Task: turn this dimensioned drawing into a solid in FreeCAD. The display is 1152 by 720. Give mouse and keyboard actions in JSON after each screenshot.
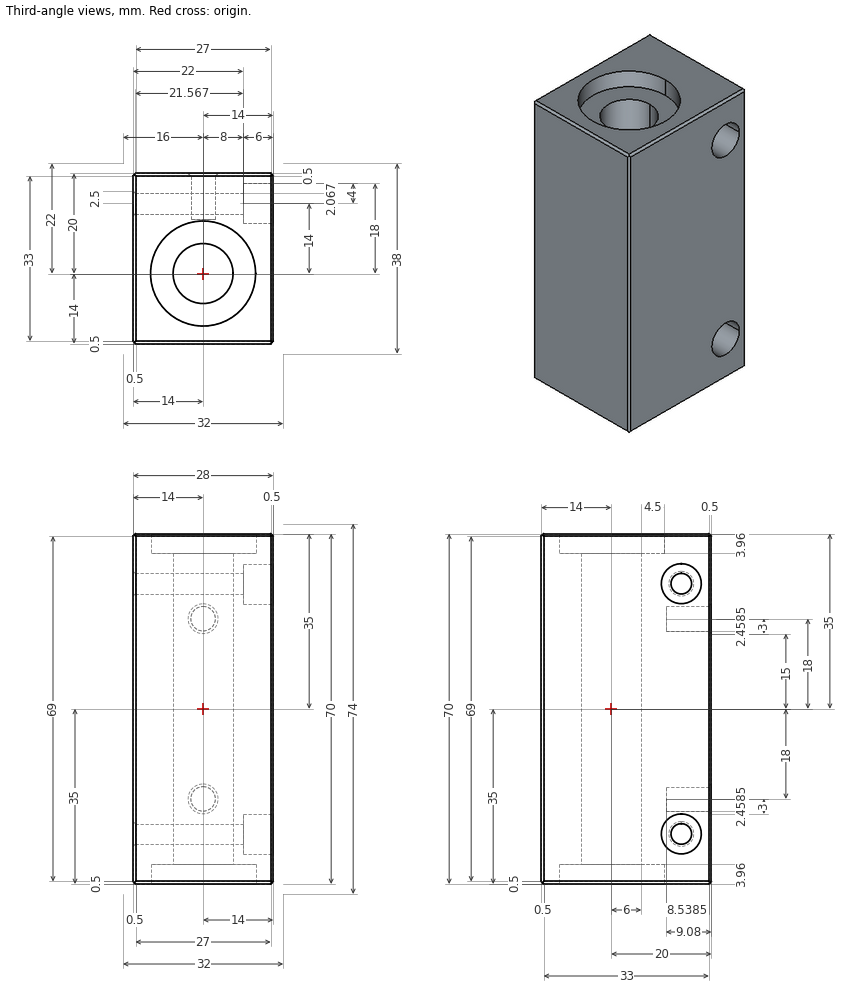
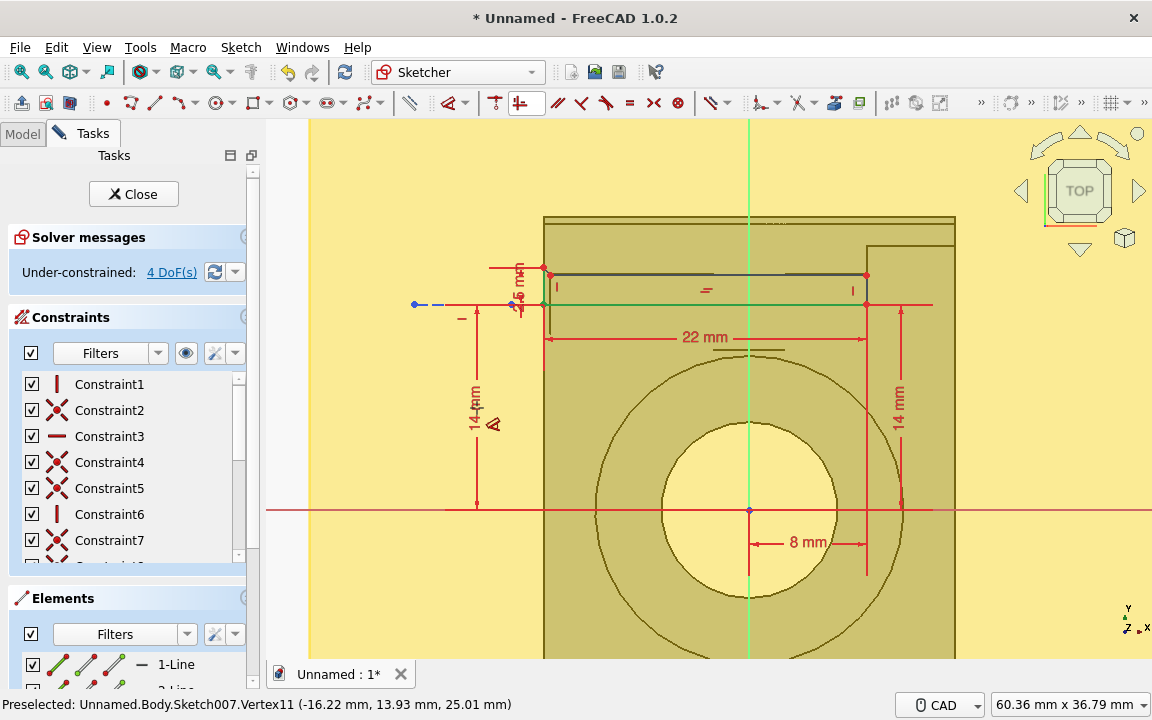
{"action": "scroll", "coordinate": [867, 293], "scroll_direction": "up", "scroll_amount": 2}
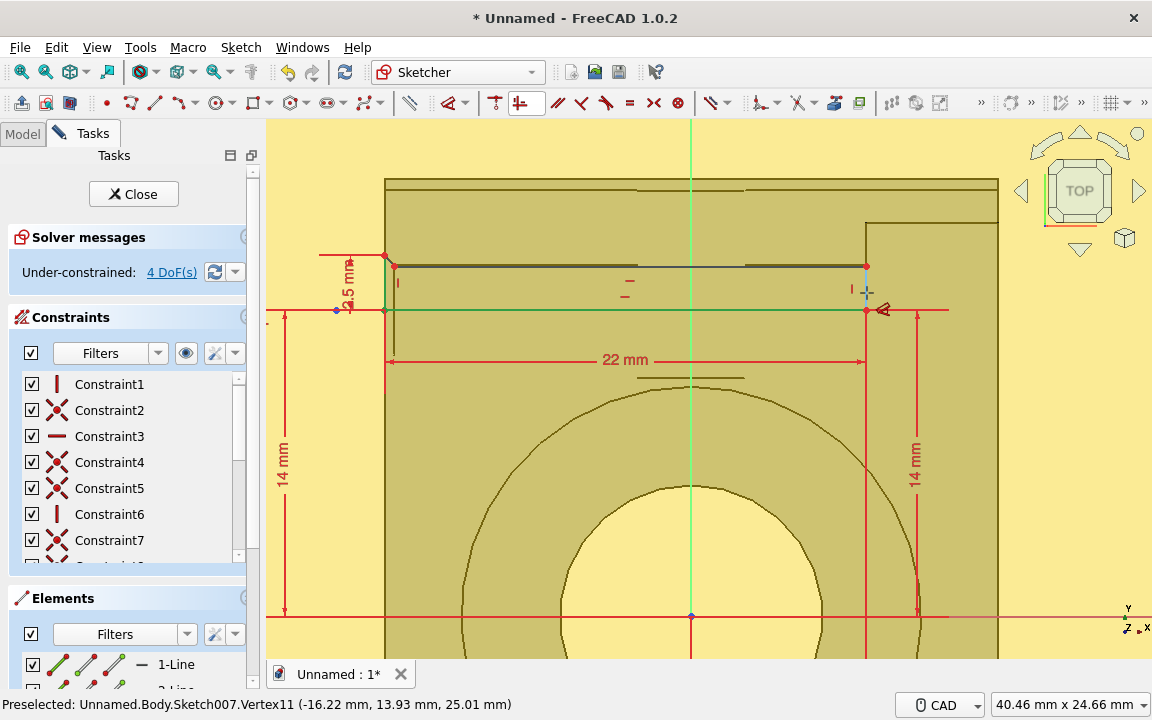
{"action": "left_click", "coordinate": [866, 293]}
{"action": "left_click", "coordinate": [900, 288]}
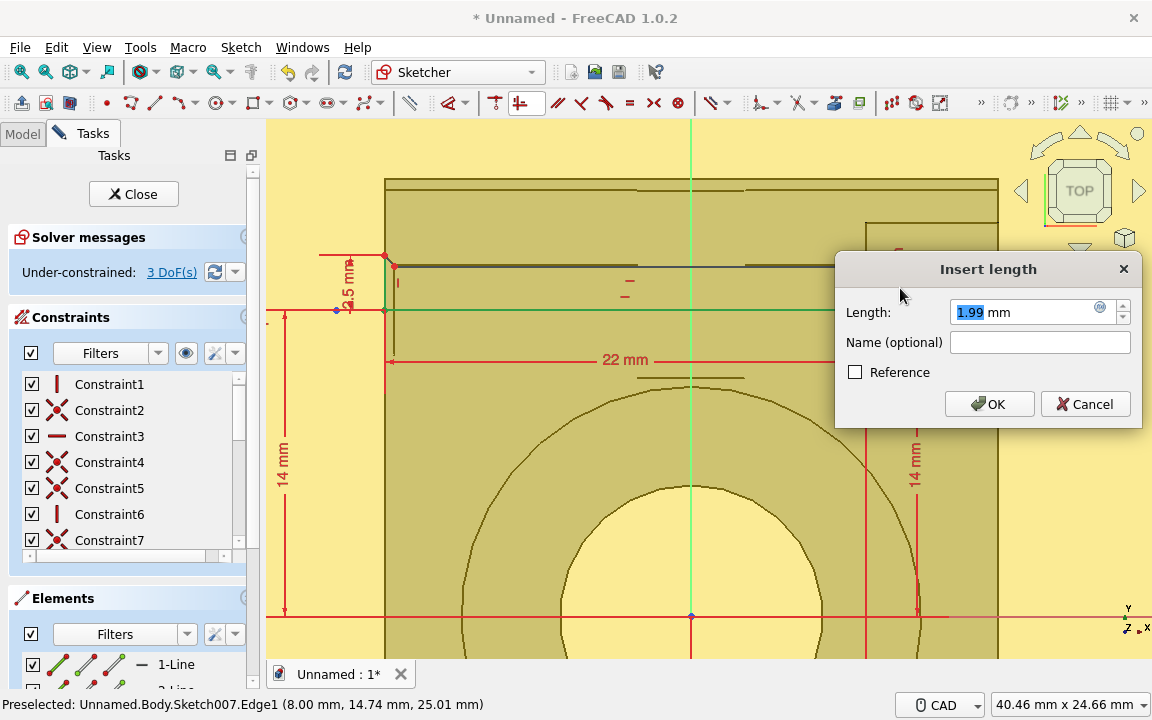
{"action": "type", "text": "2.067"}
{"action": "key", "text": "Return"}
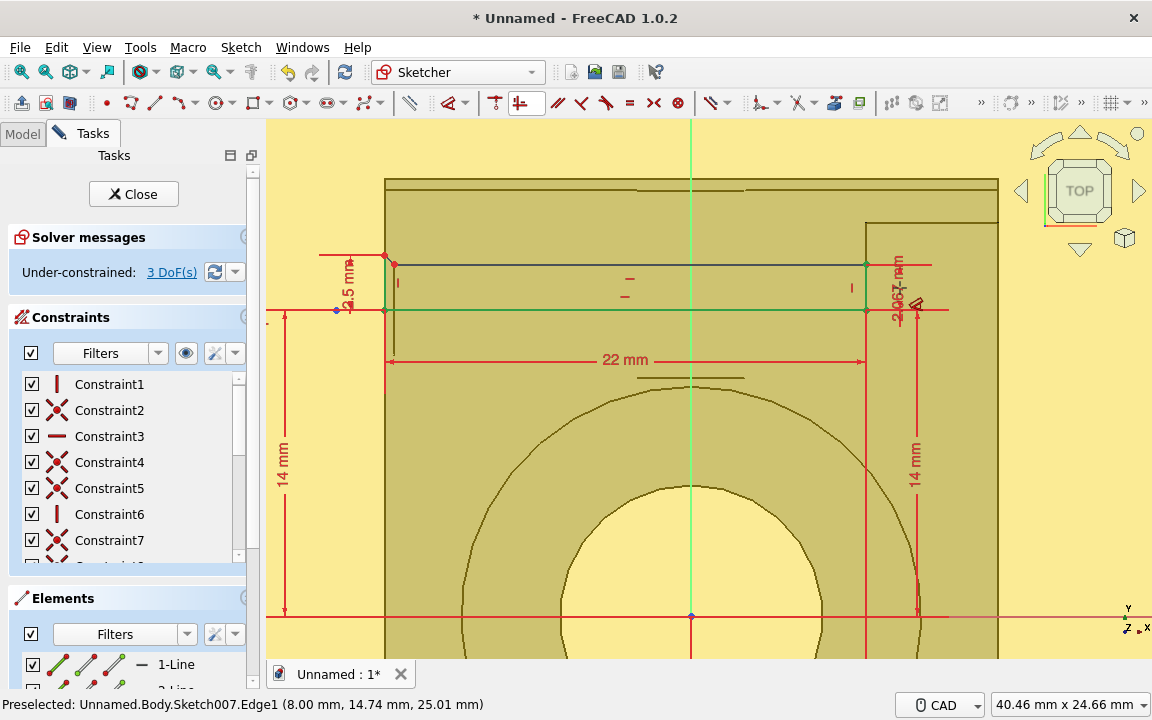
{"action": "left_click", "coordinate": [725, 265]}
{"action": "left_click", "coordinate": [631, 231]}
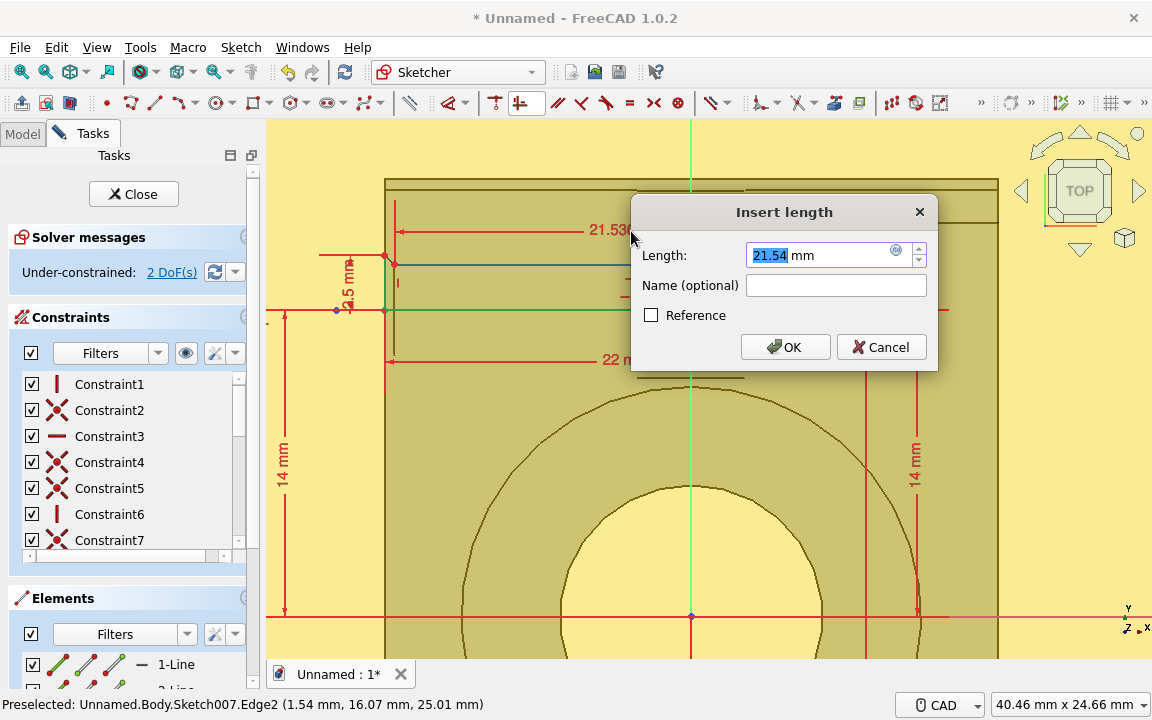
{"action": "type", "text": "21.567"}
{"action": "key", "text": "Return"}
{"action": "key", "text": "Escape"}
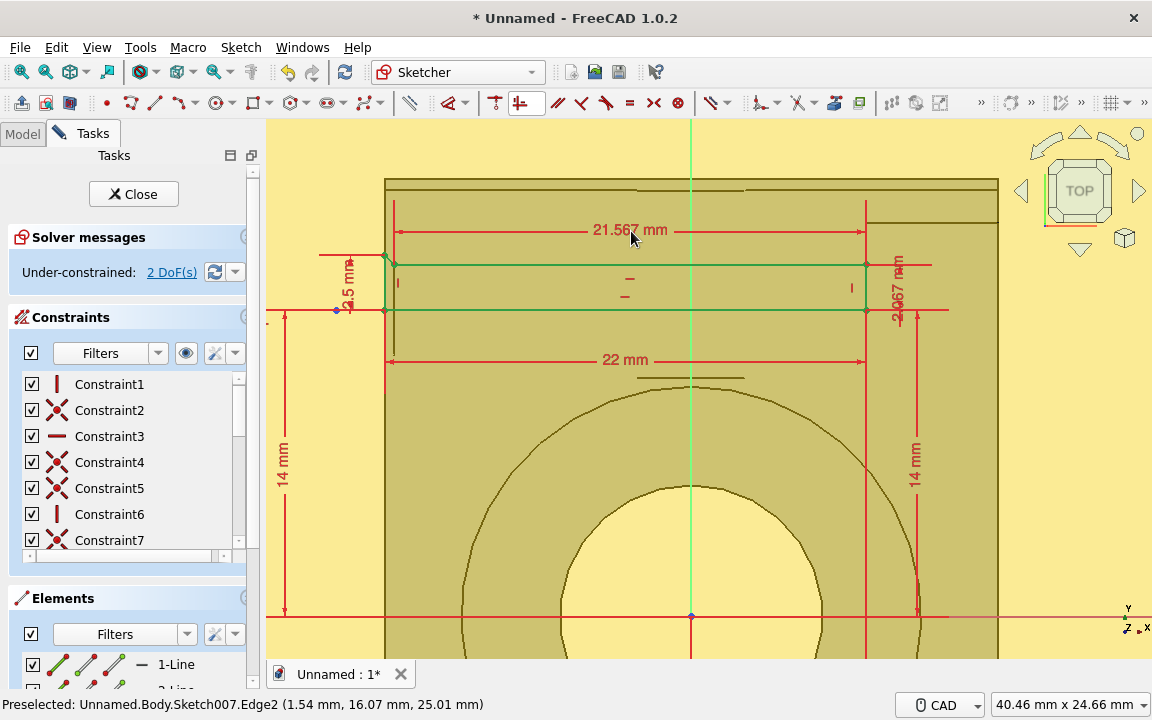
{"action": "left_click", "coordinate": [134, 194]}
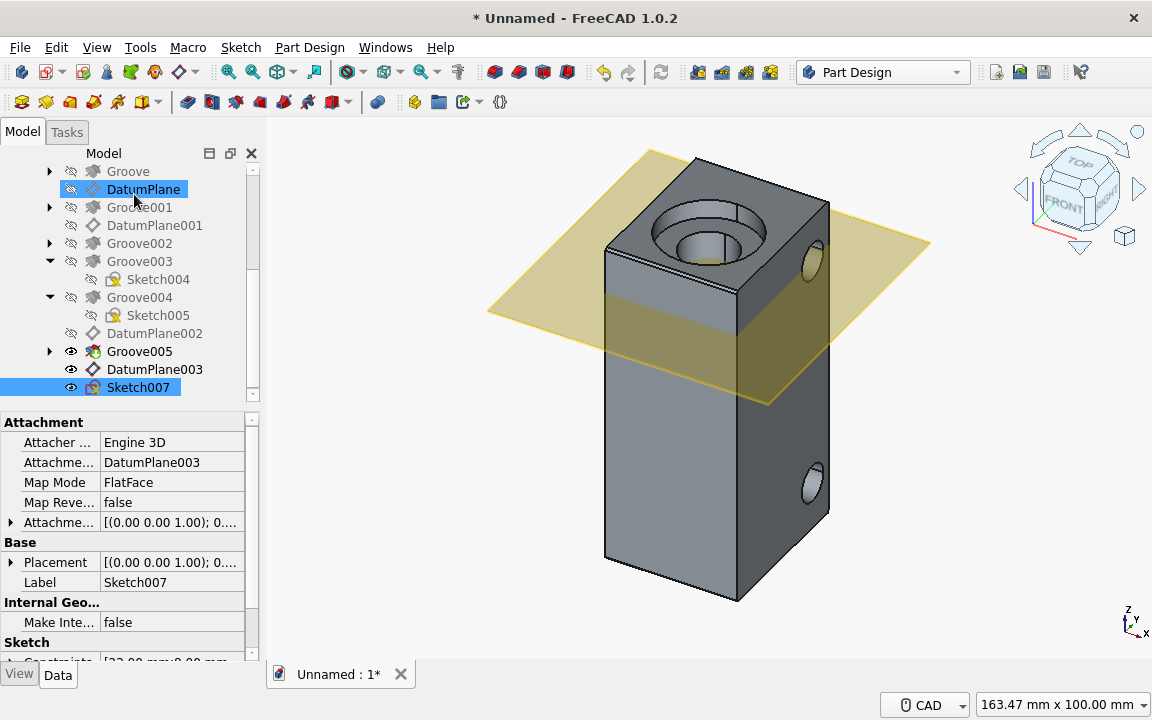
{"action": "left_click", "coordinate": [236, 102]}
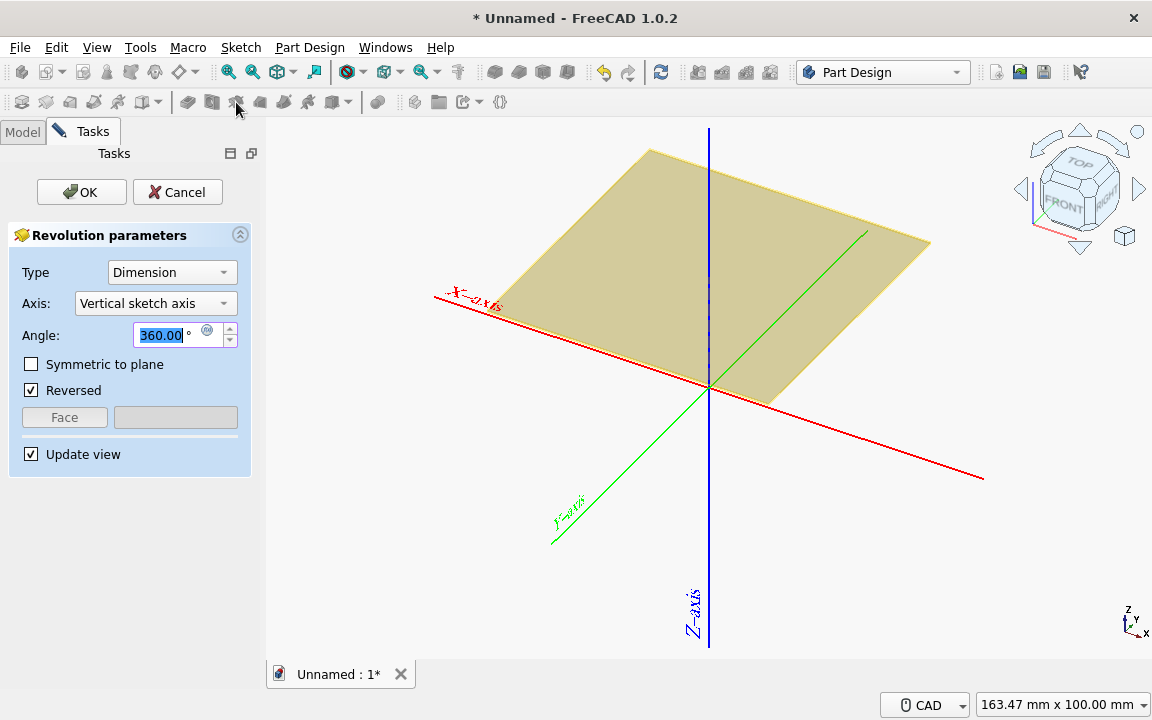
{"action": "left_click", "coordinate": [156, 304]}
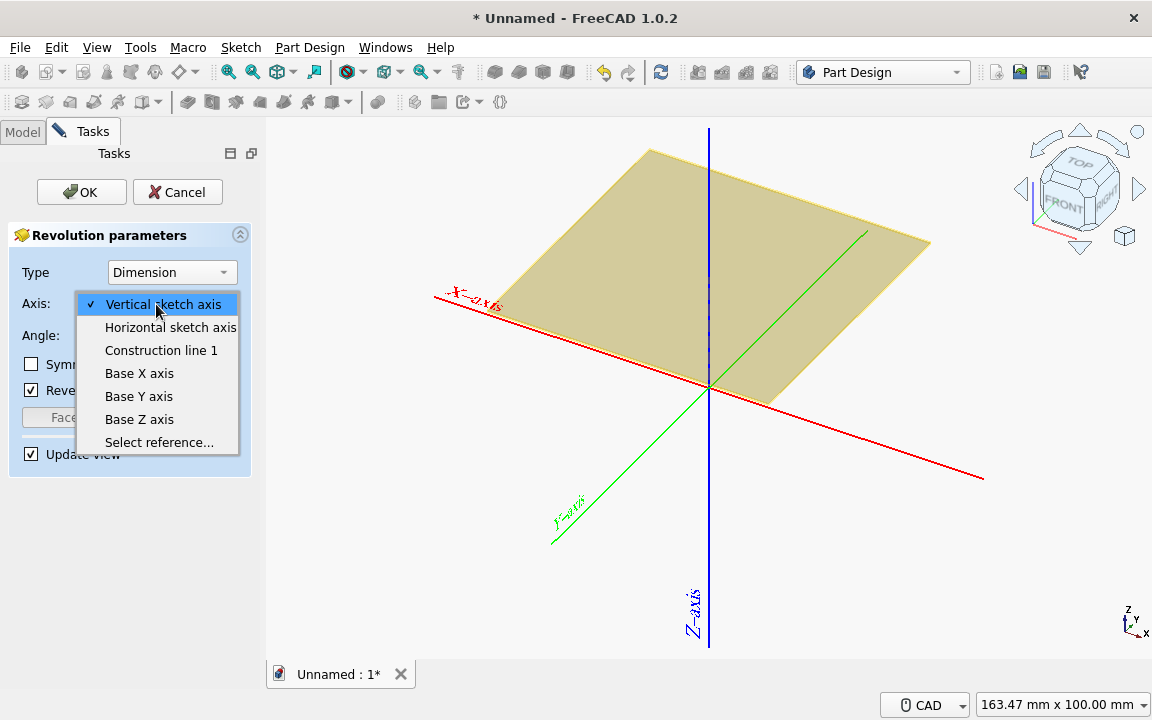
{"action": "left_click", "coordinate": [156, 350]}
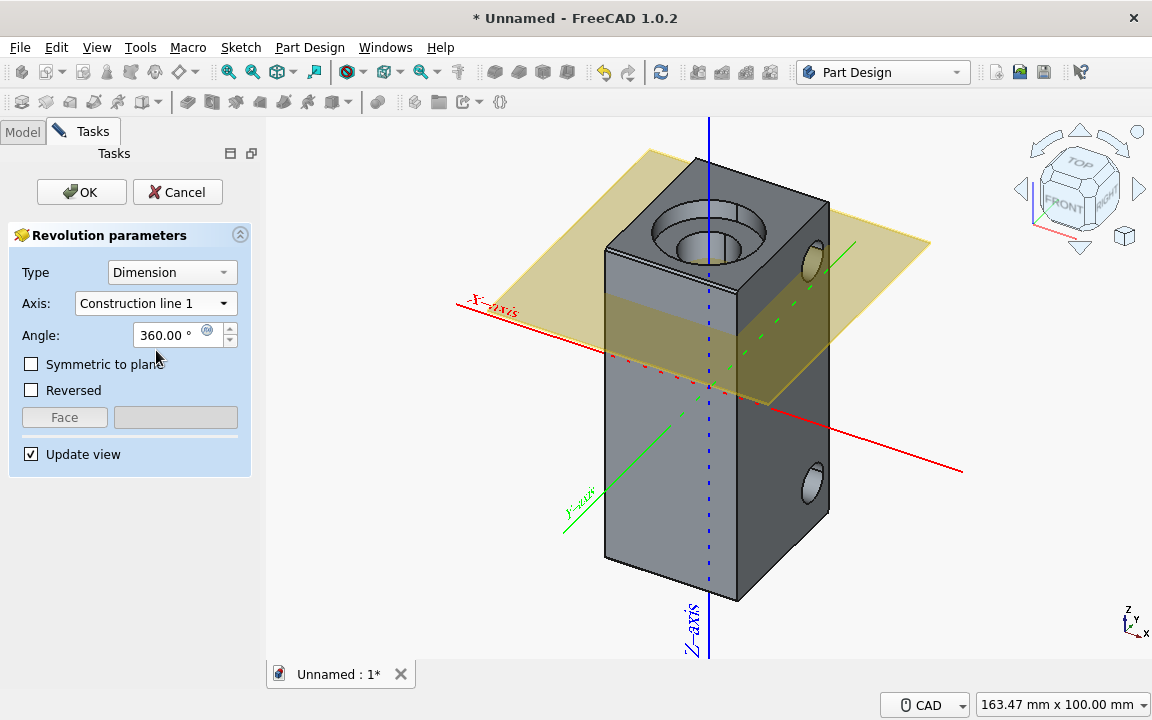
{"action": "left_click", "coordinate": [82, 192]}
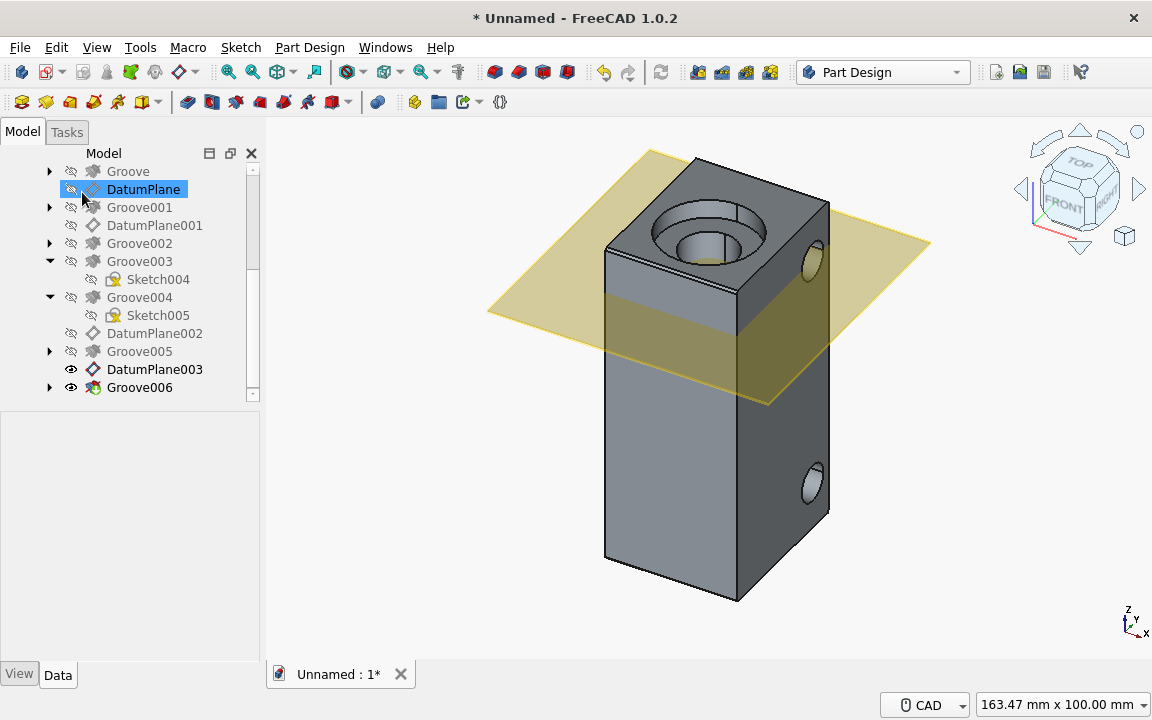
{"action": "left_click", "coordinate": [116, 369]}
{"action": "key", "text": "space"}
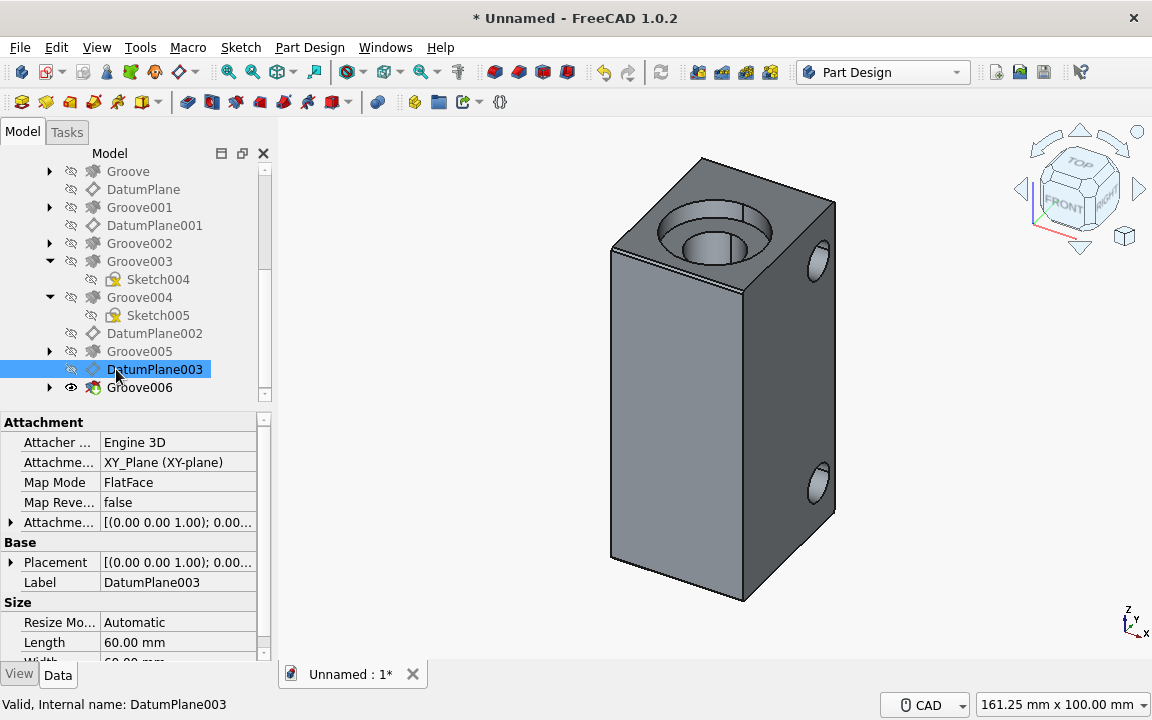
{"action": "left_click", "coordinate": [318, 619]}